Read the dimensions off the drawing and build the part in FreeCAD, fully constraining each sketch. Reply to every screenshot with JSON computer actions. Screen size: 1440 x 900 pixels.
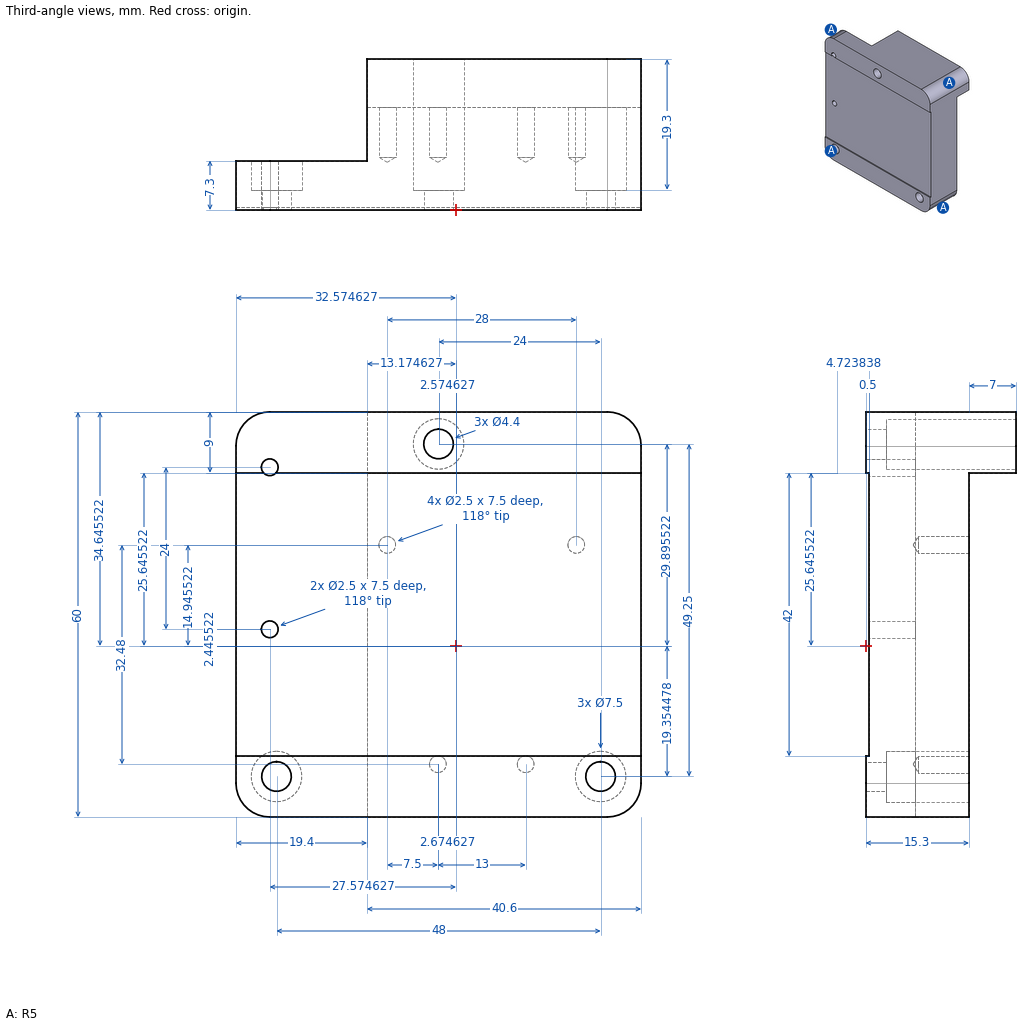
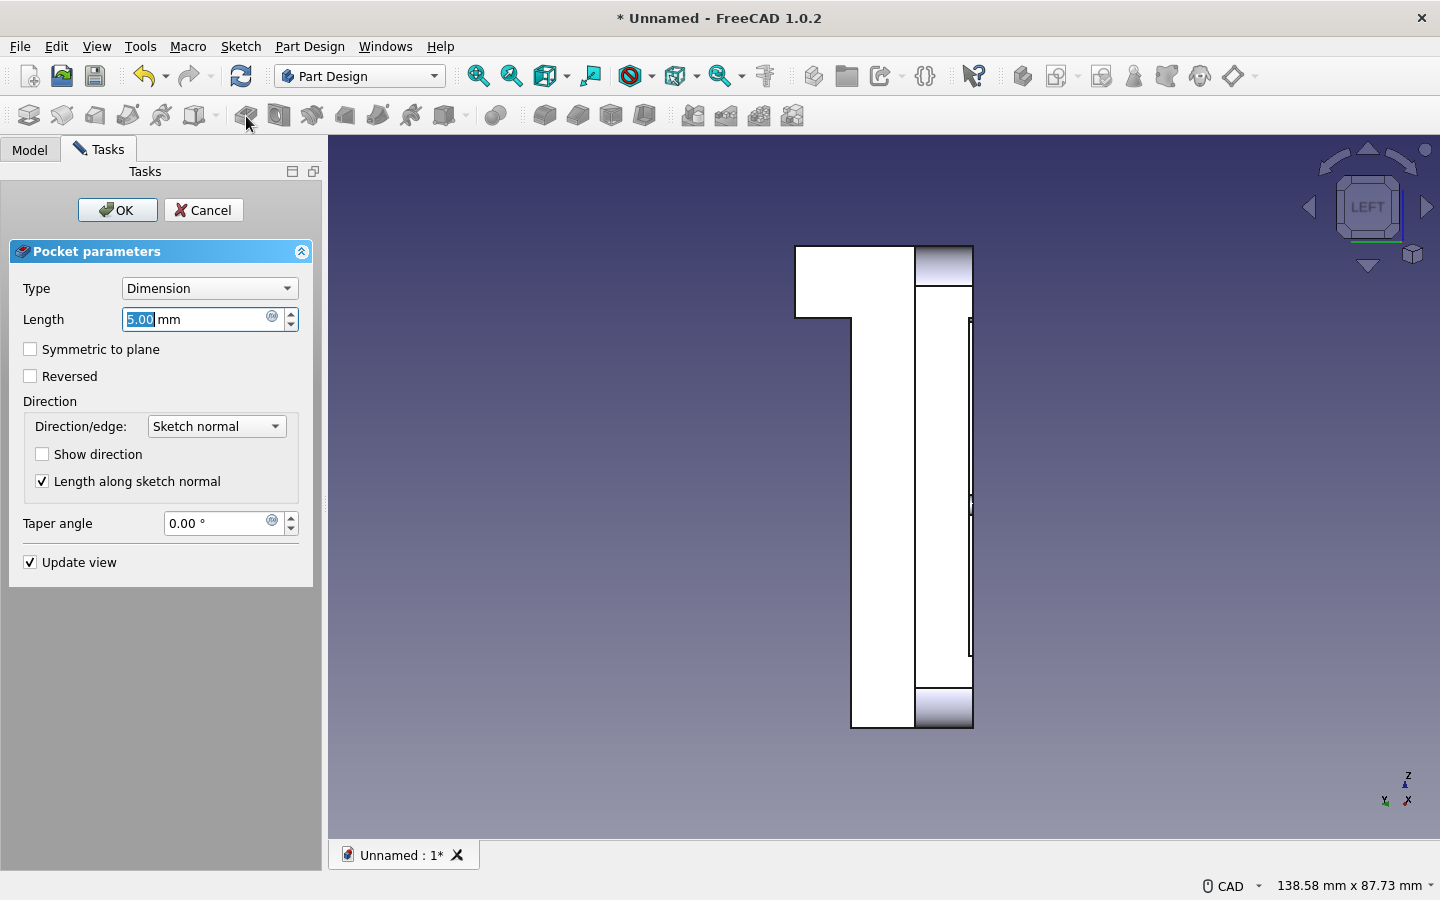
{"action": "left_click", "coordinate": [210, 288]}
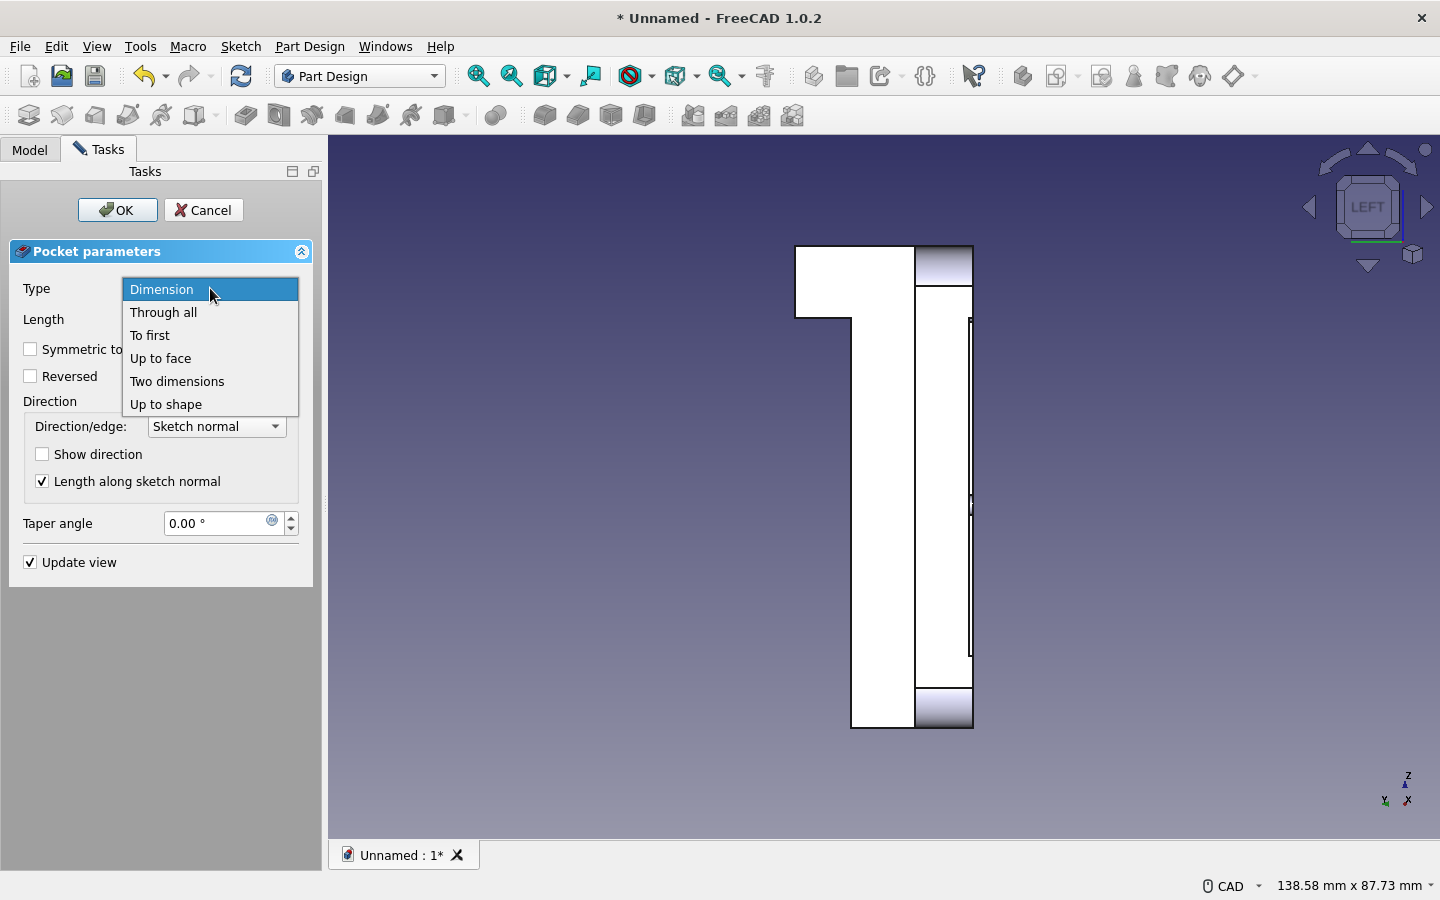
{"action": "left_click", "coordinate": [208, 312]}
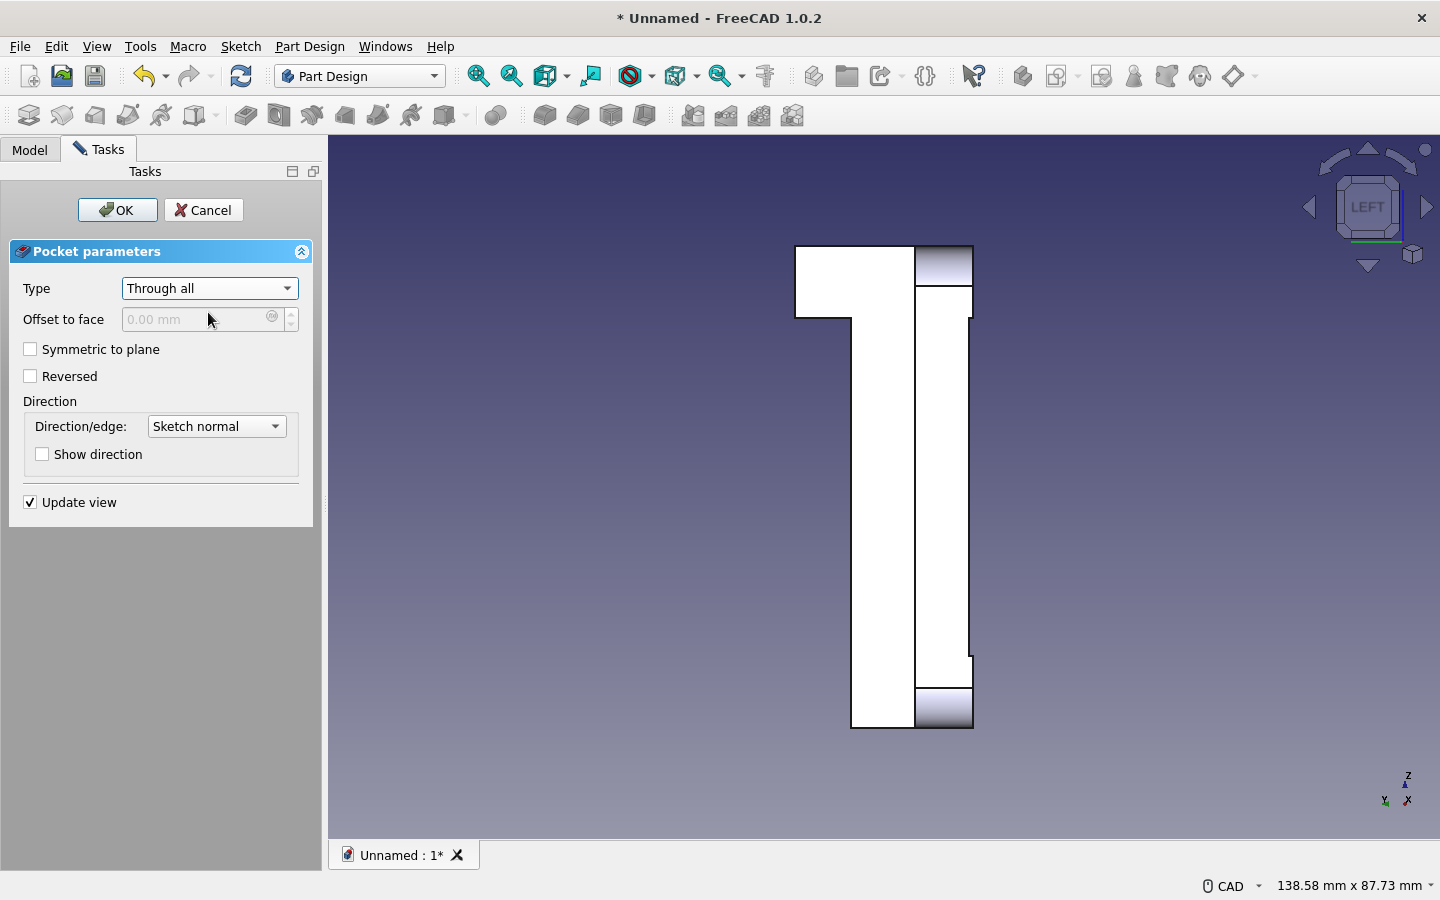
{"action": "left_click", "coordinate": [118, 210]}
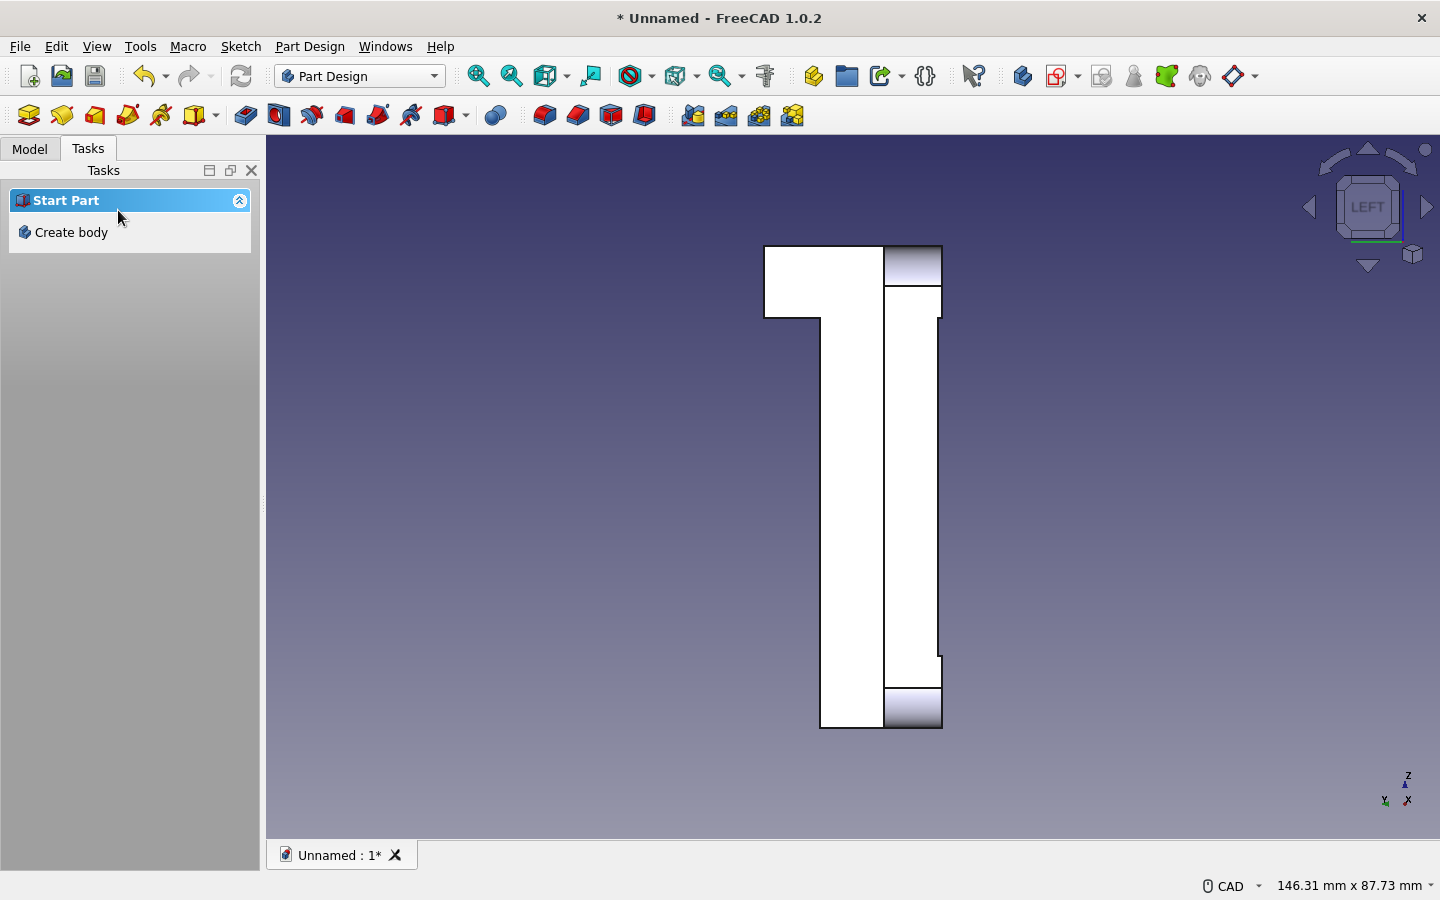
{"action": "key", "text": "4"}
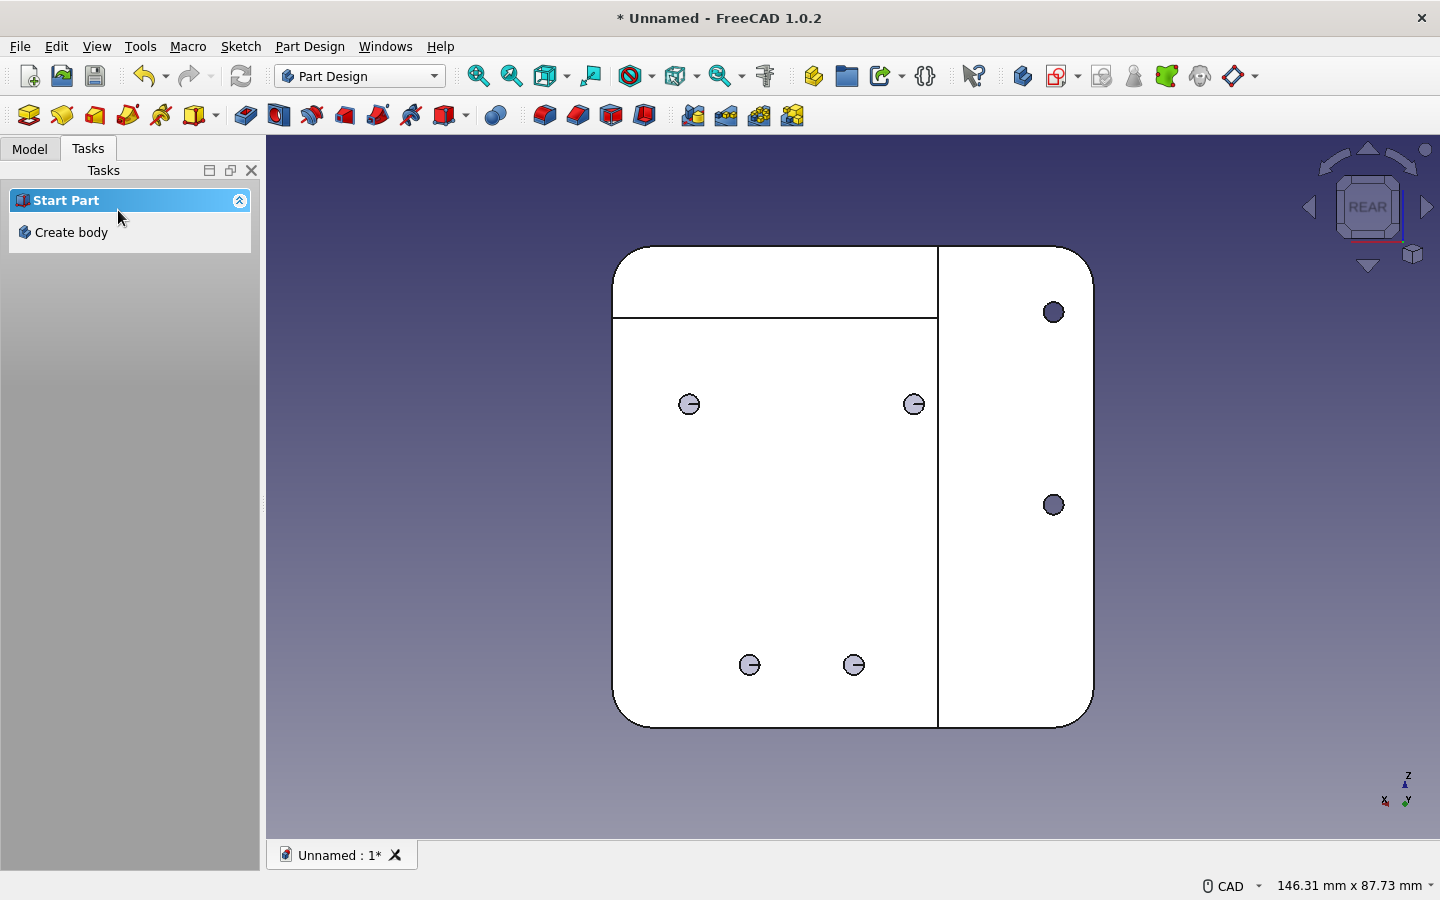
{"action": "left_click", "coordinate": [682, 281]}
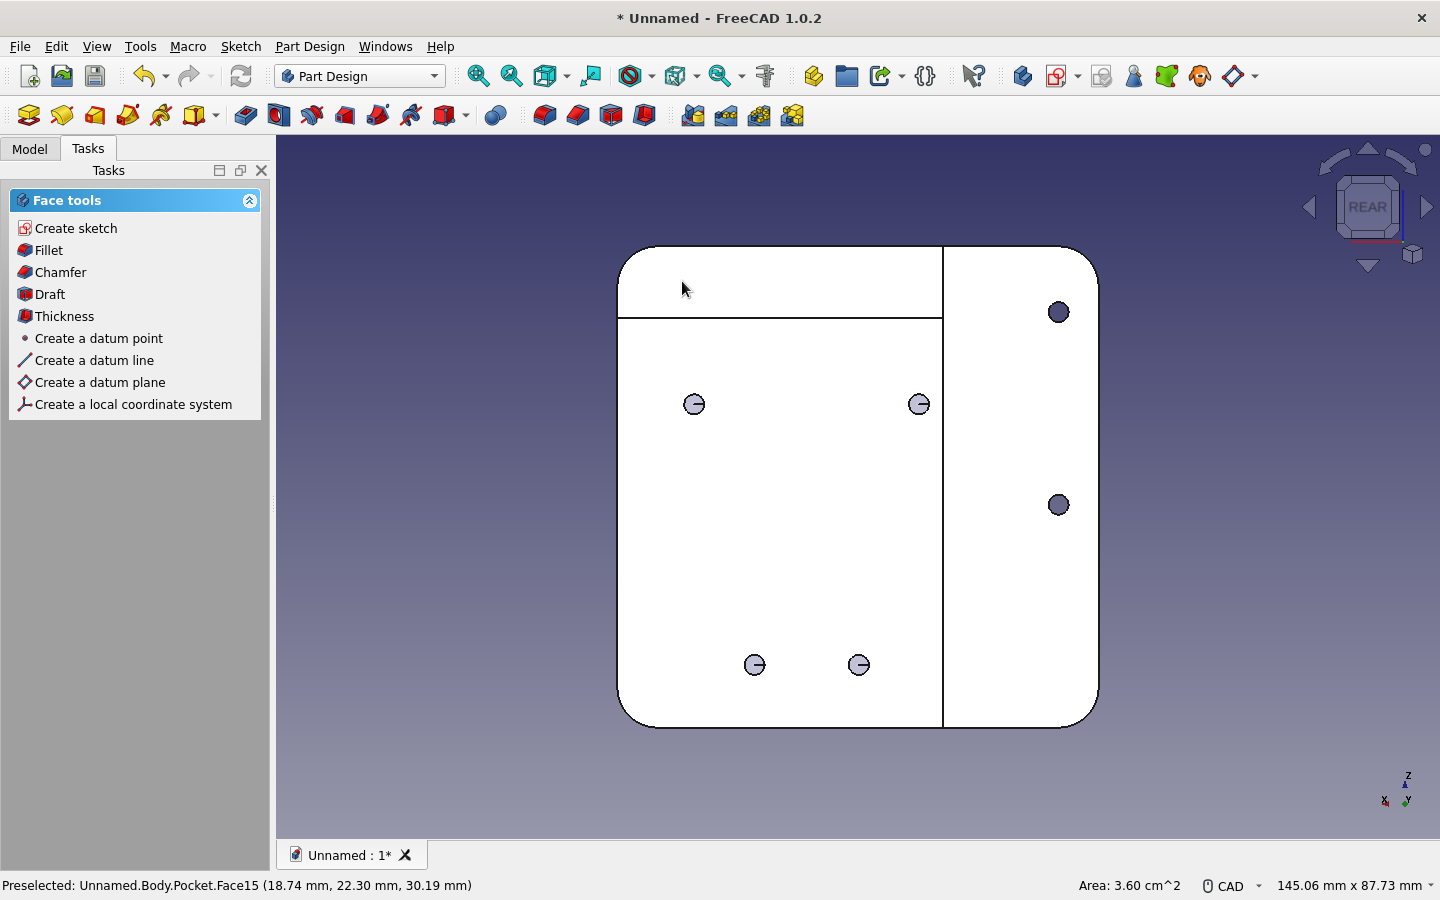
{"action": "left_click", "coordinate": [1056, 76]}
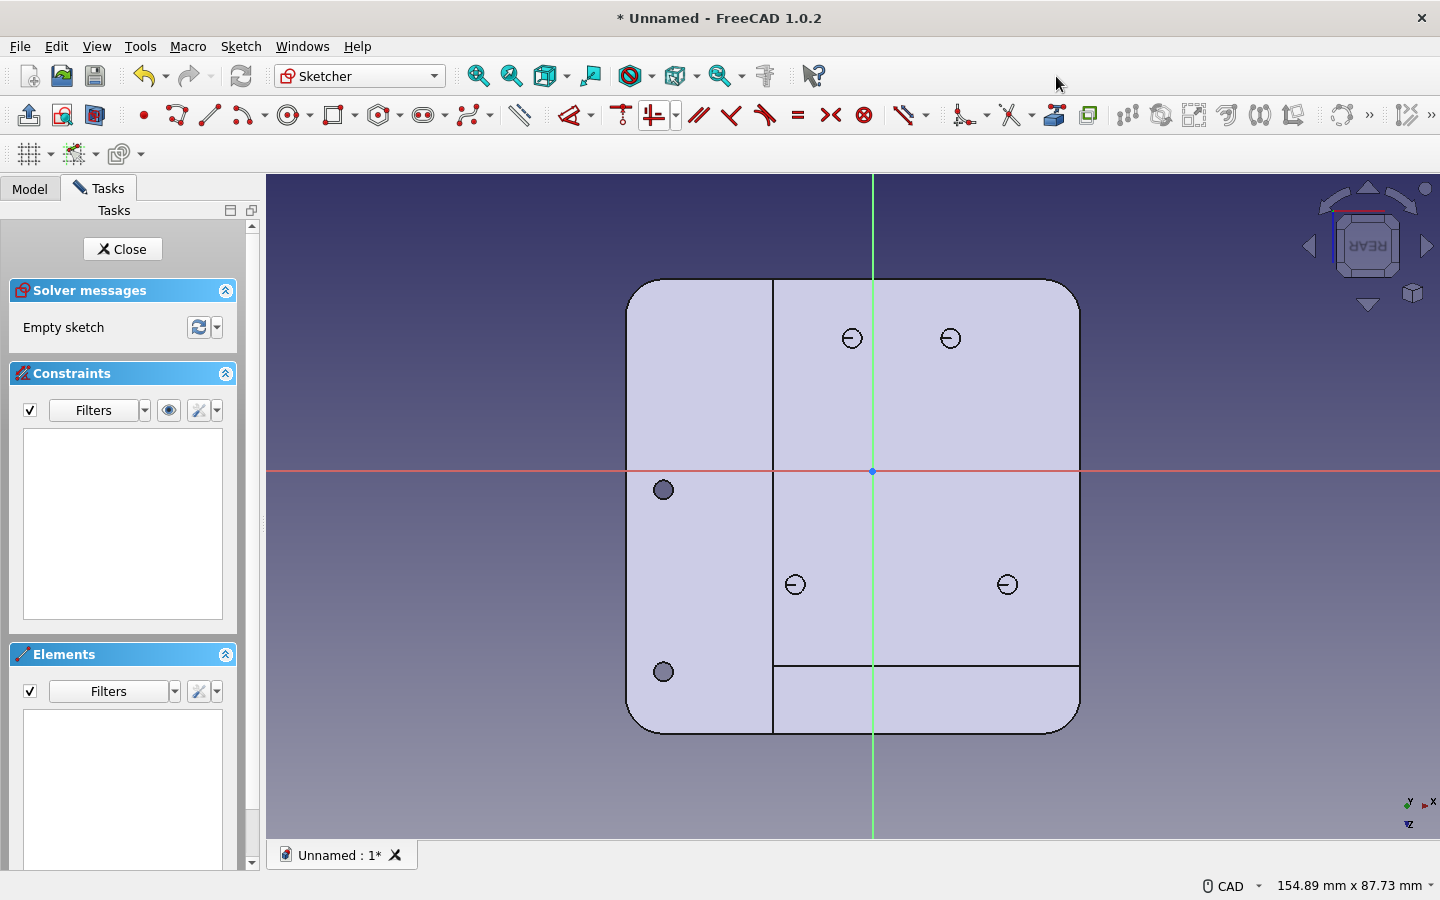
{"action": "key", "text": "g c"}